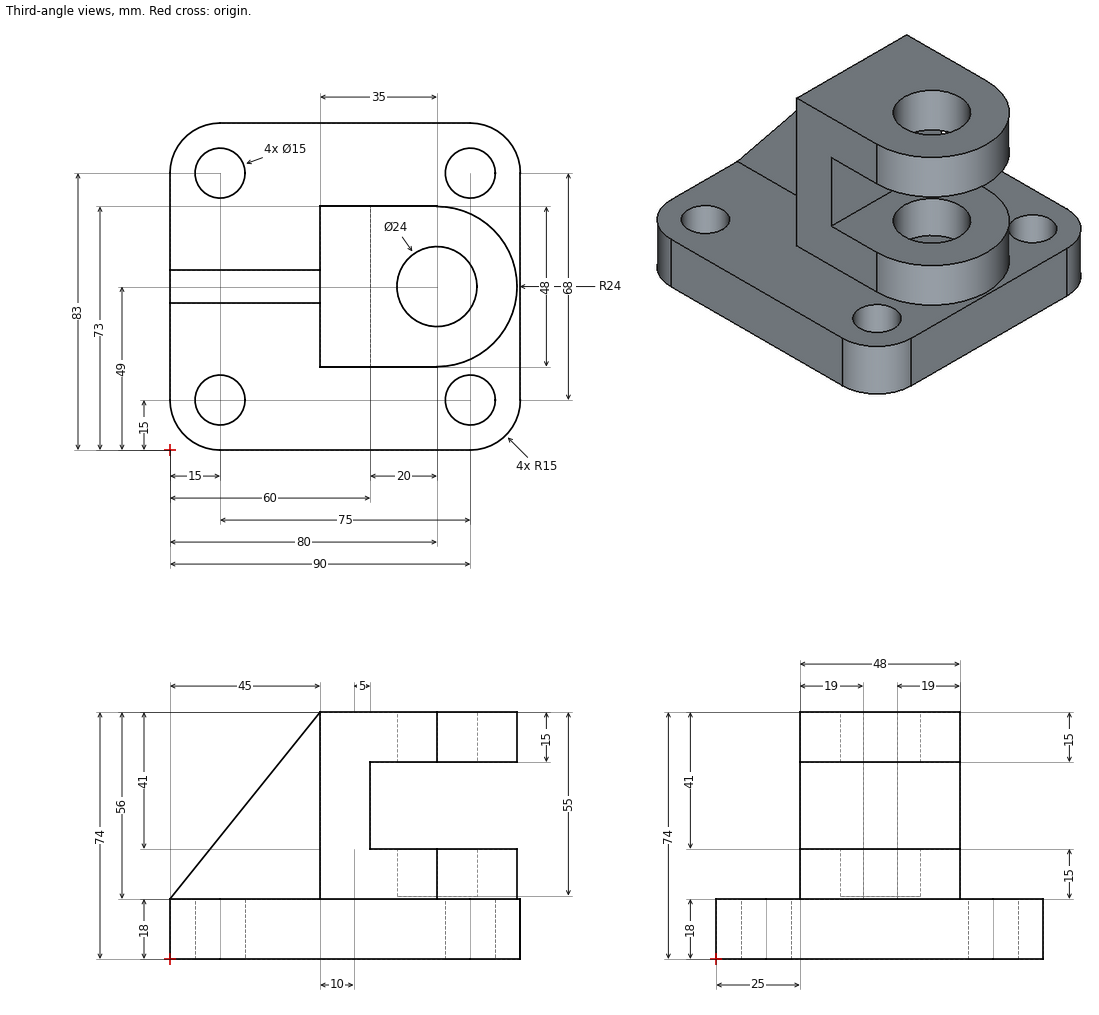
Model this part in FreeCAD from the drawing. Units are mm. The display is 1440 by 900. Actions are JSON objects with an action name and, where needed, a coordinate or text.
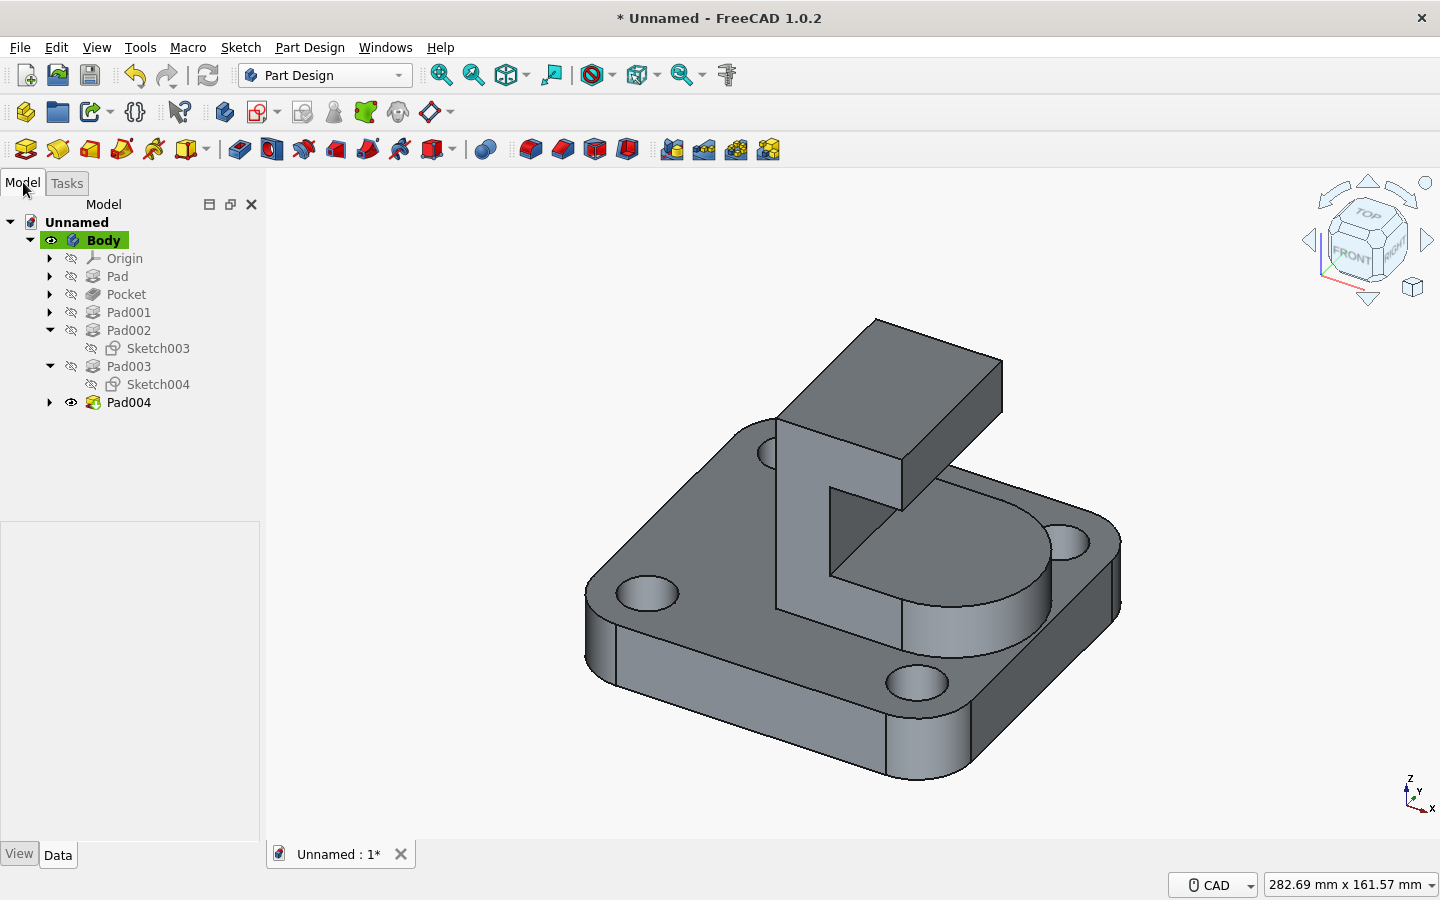
{"action": "left_click", "coordinate": [50, 258]}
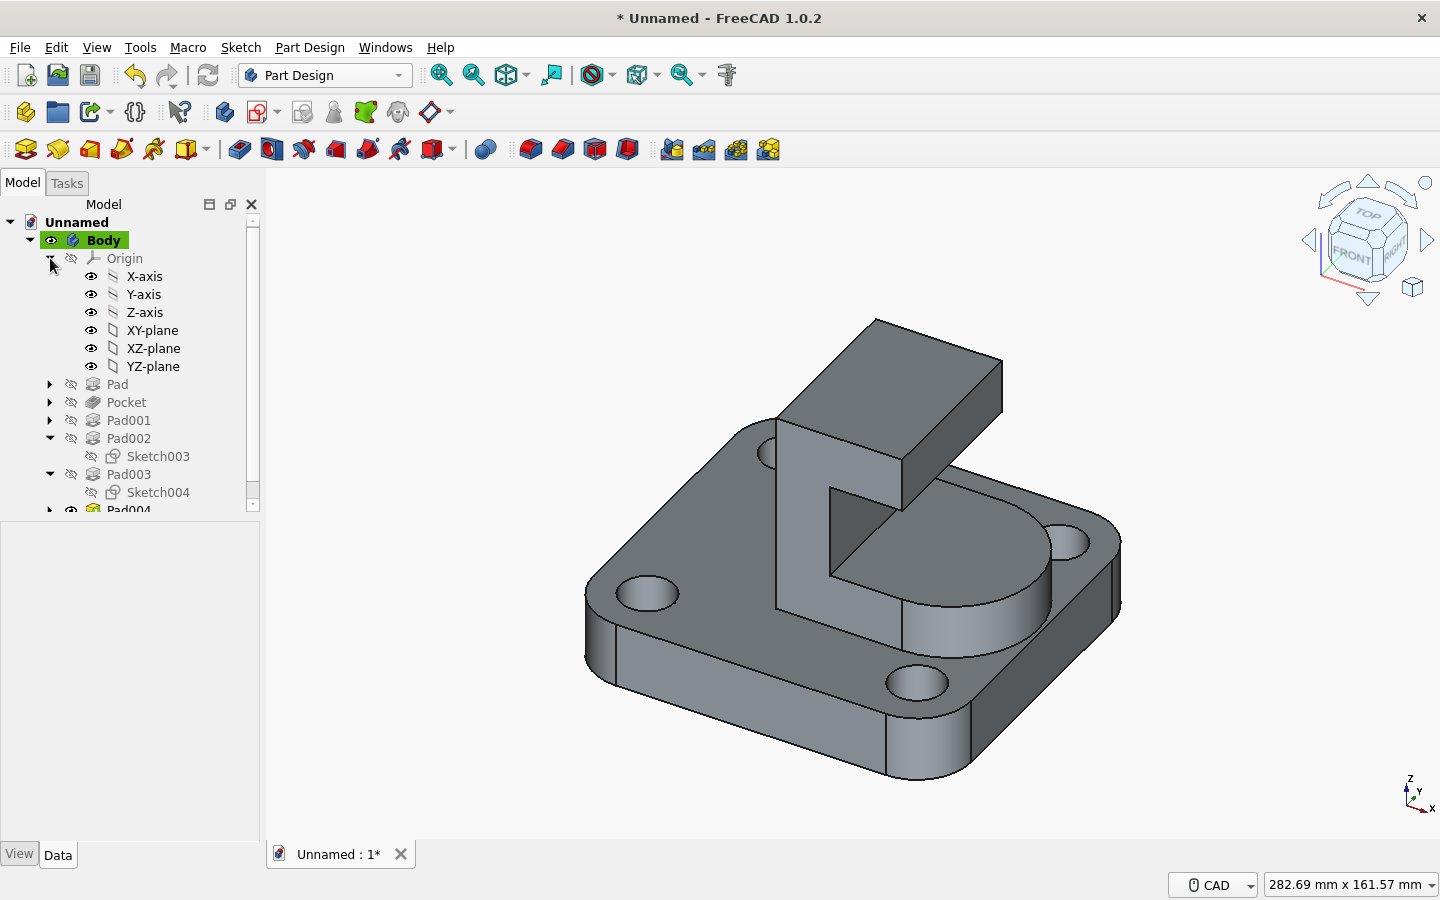
{"action": "left_click", "coordinate": [136, 330]}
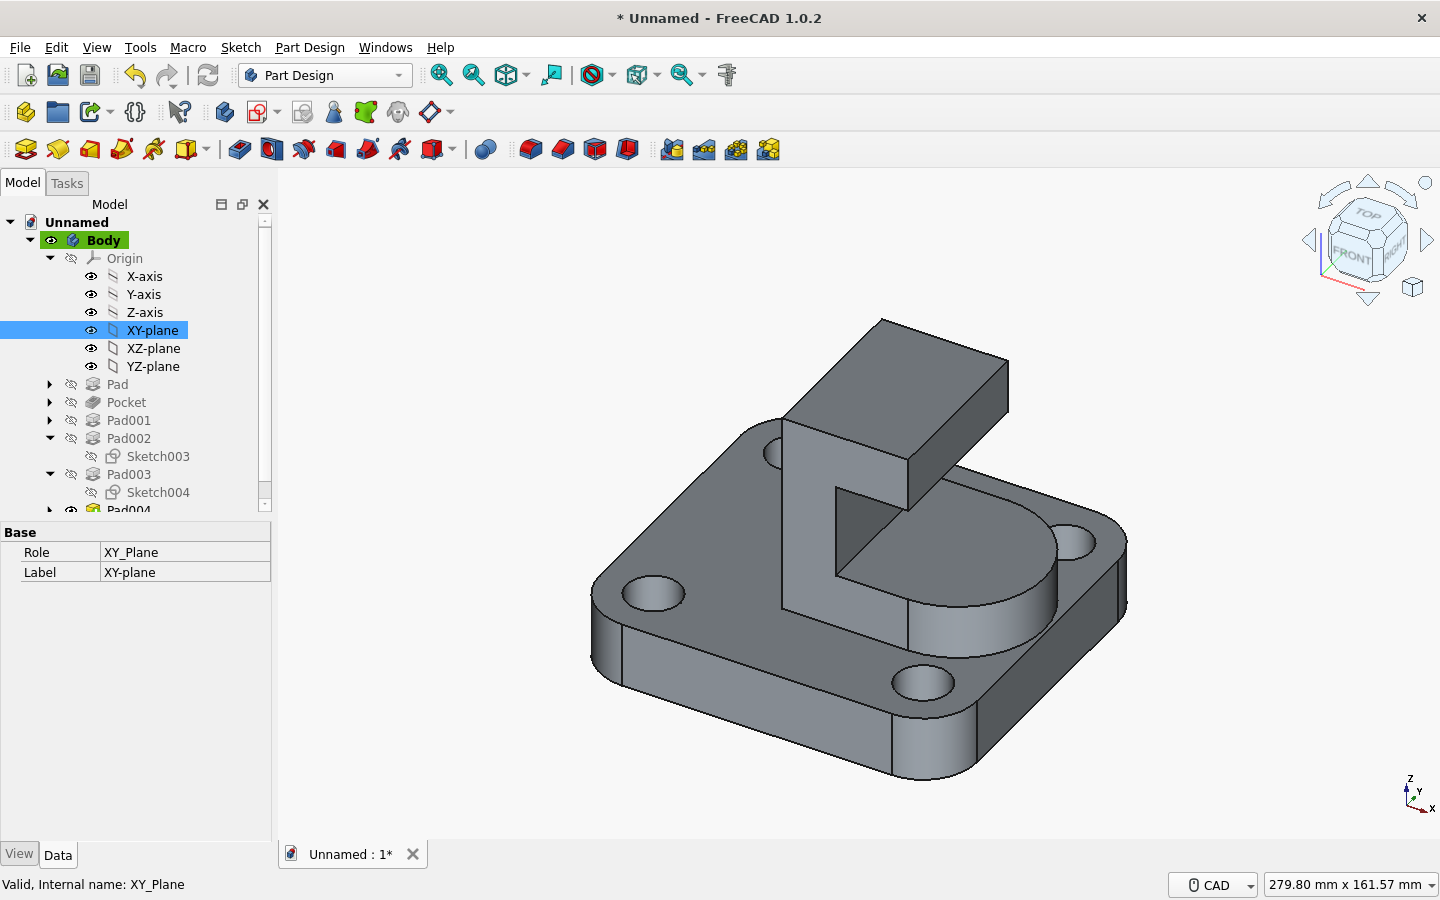
{"action": "left_click", "coordinate": [430, 112]}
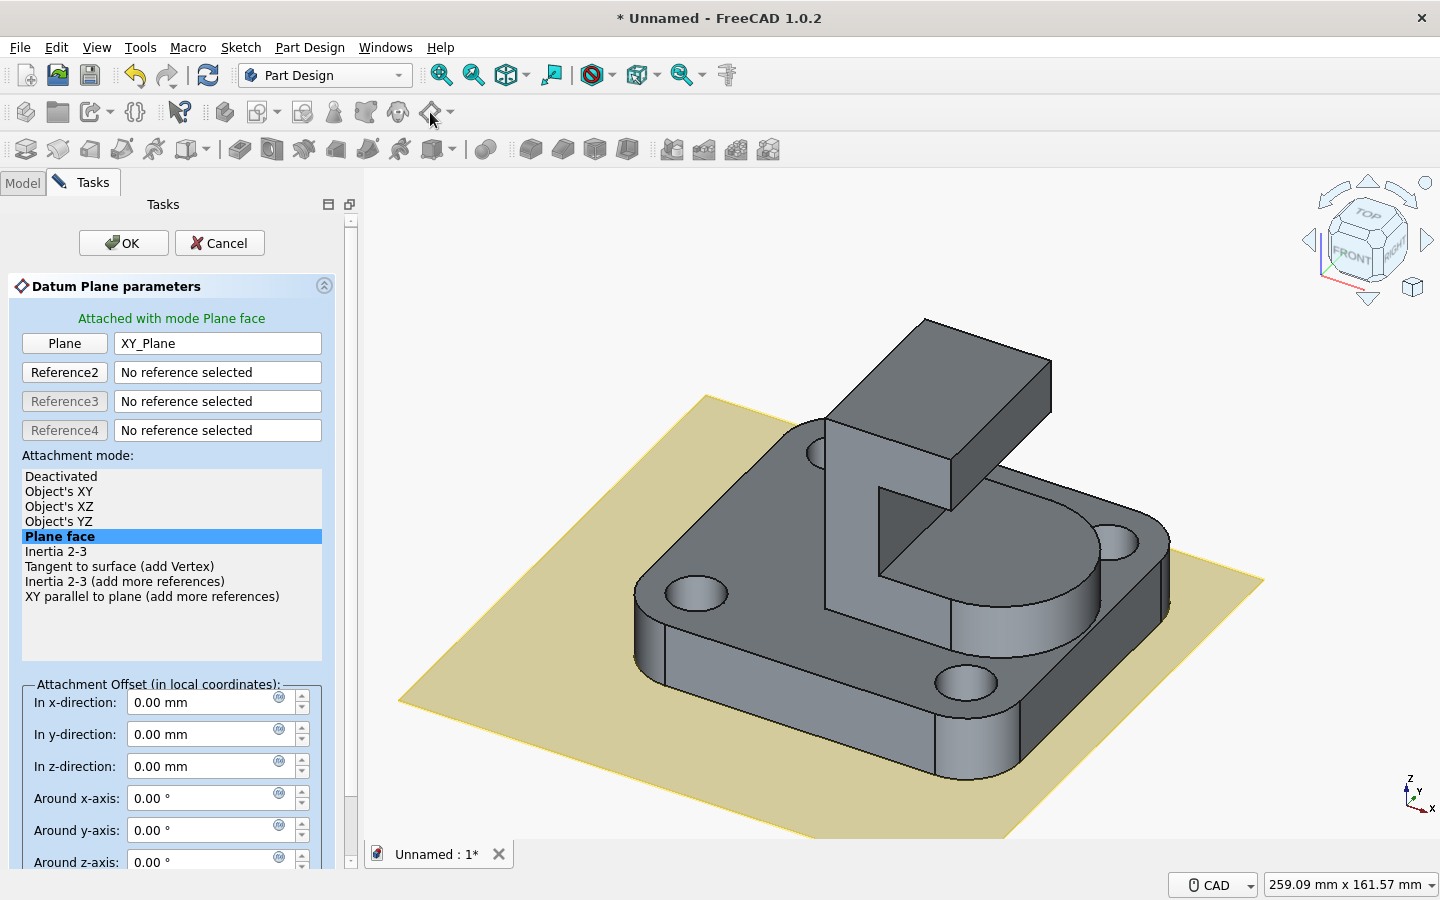
{"action": "triple_click", "coordinate": [210, 766]}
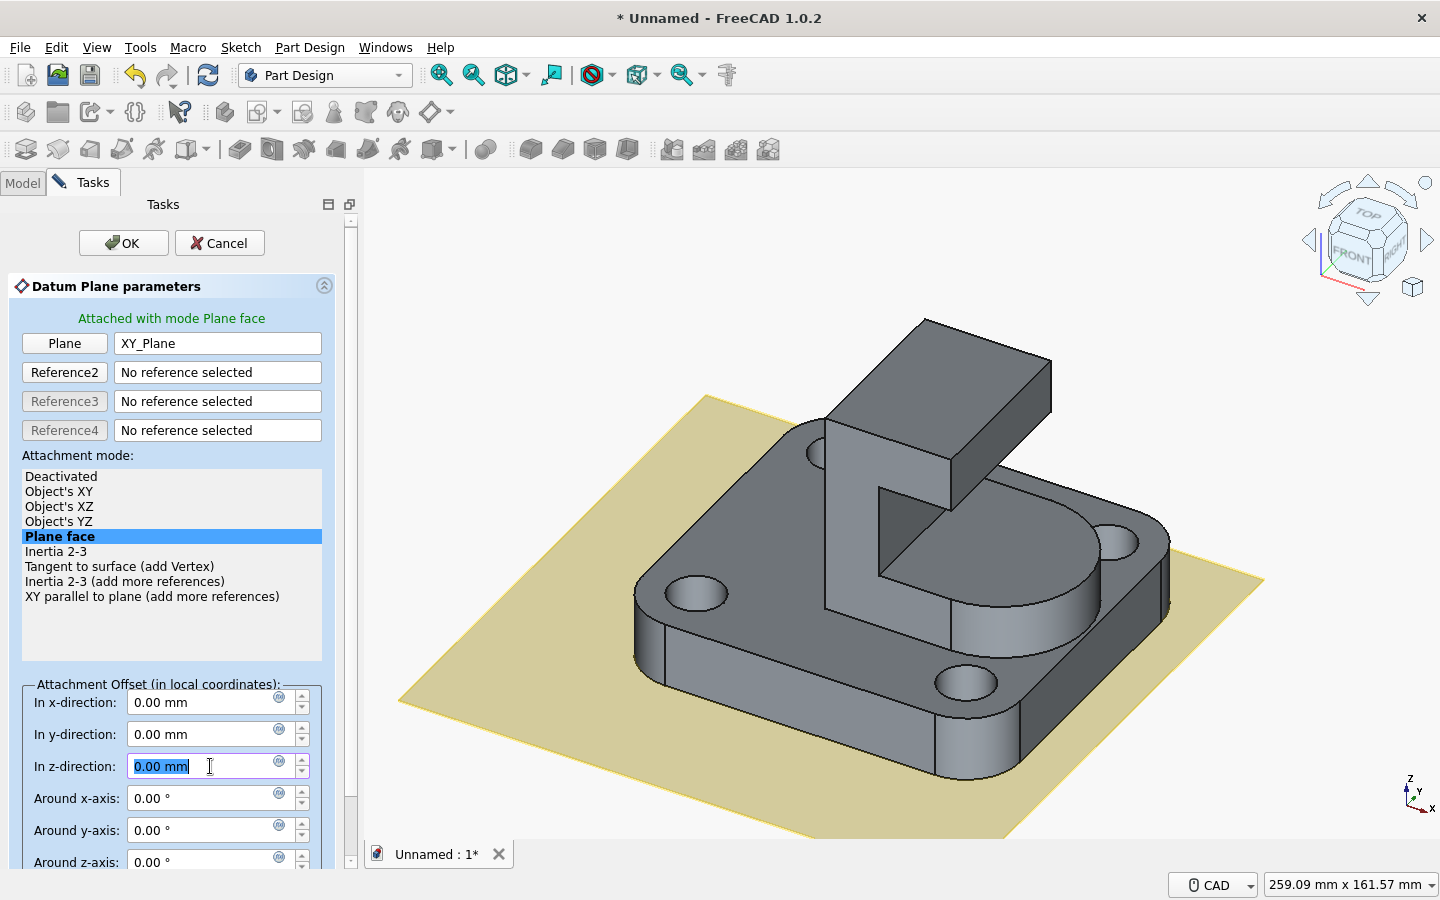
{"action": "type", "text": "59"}
{"action": "key", "text": "Tab"}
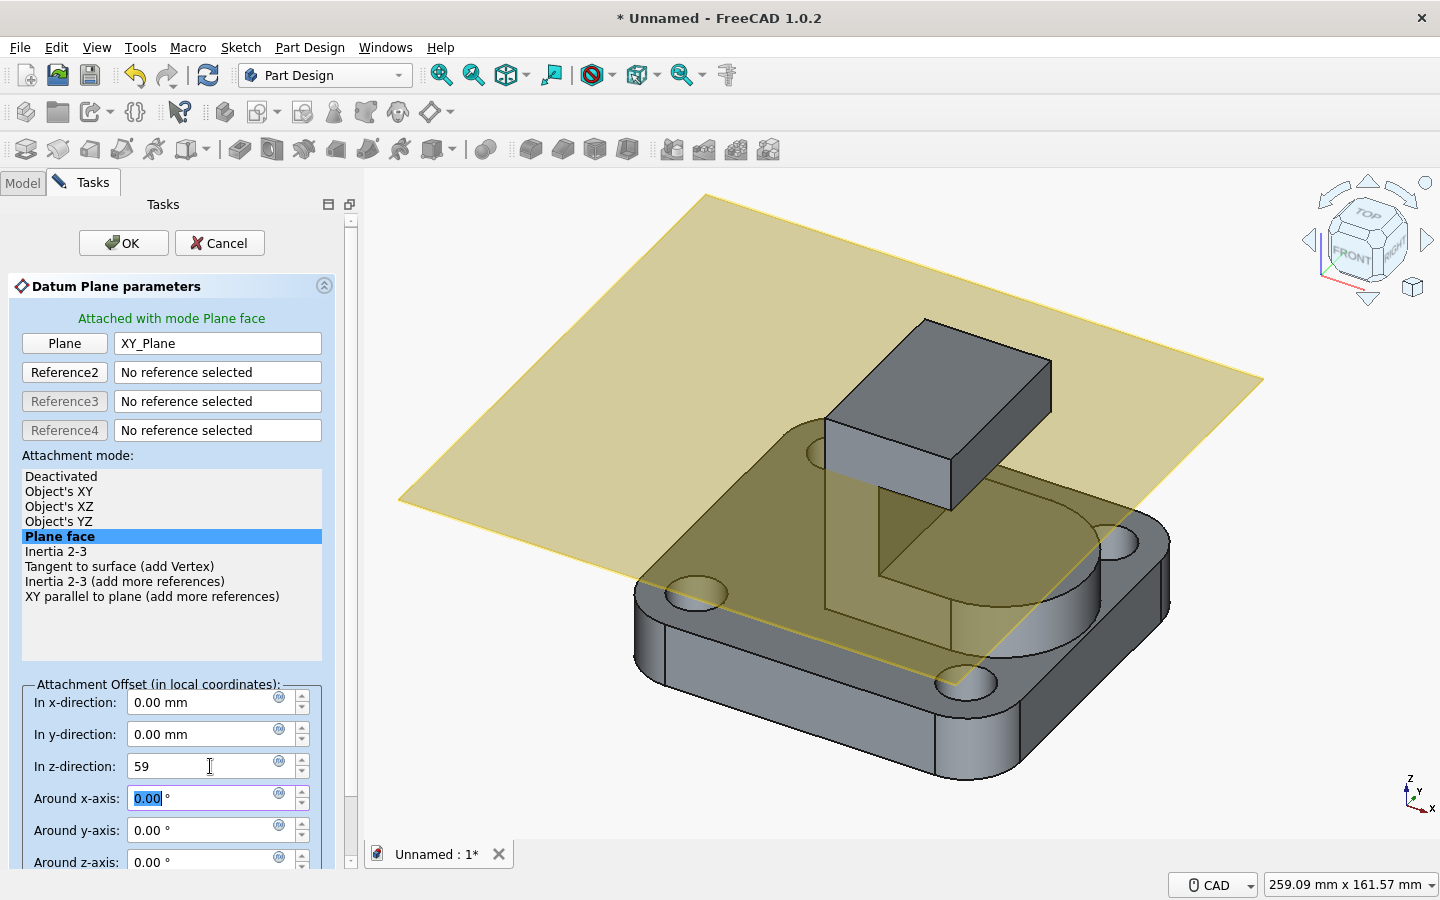
{"action": "left_click", "coordinate": [124, 243]}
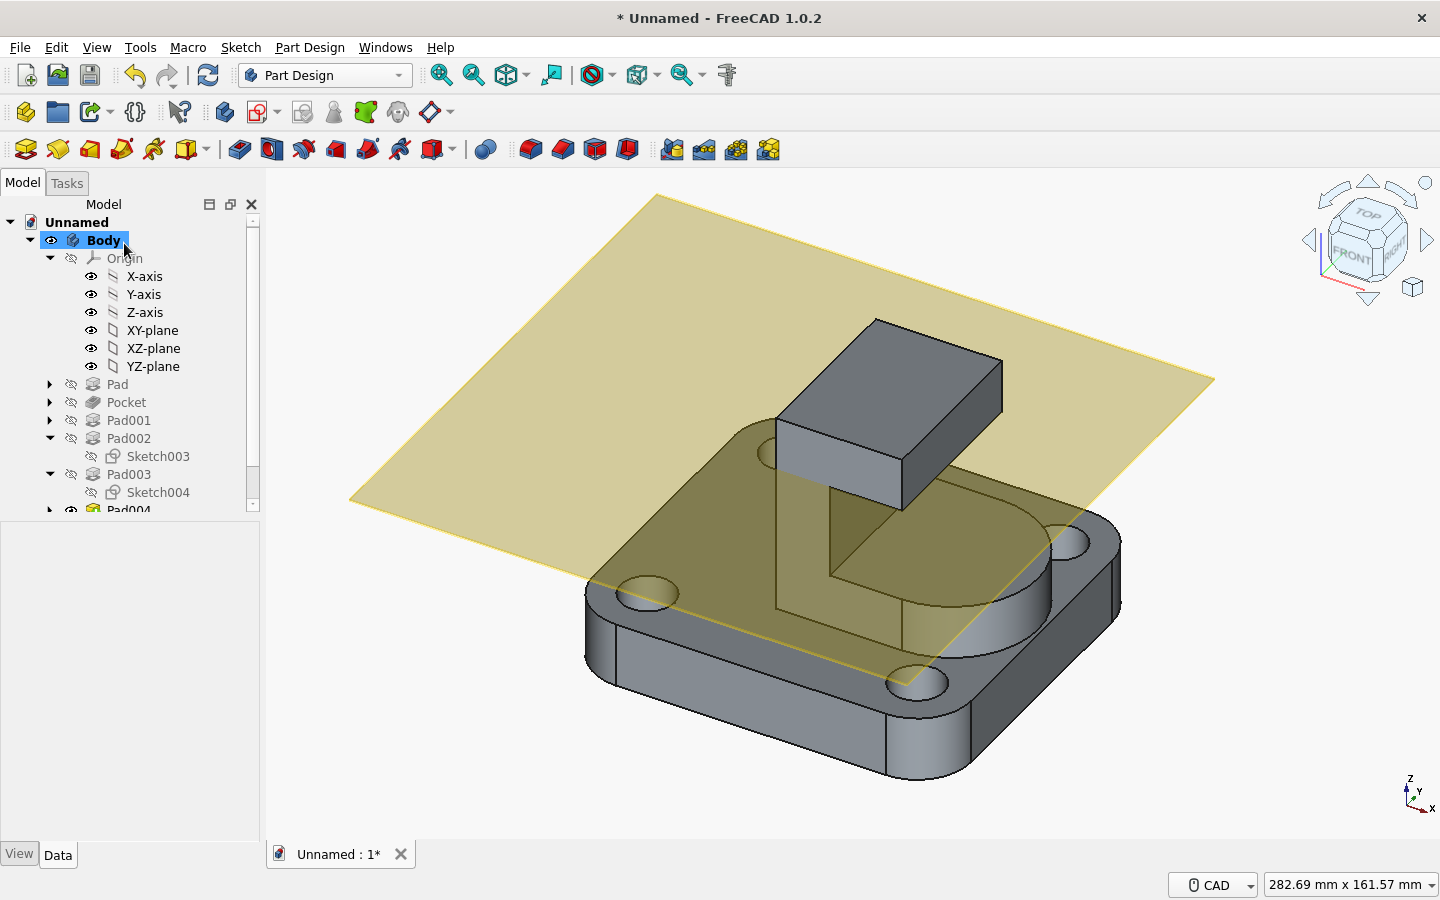
{"action": "scroll", "coordinate": [100, 362], "scroll_direction": "down", "scroll_amount": 3}